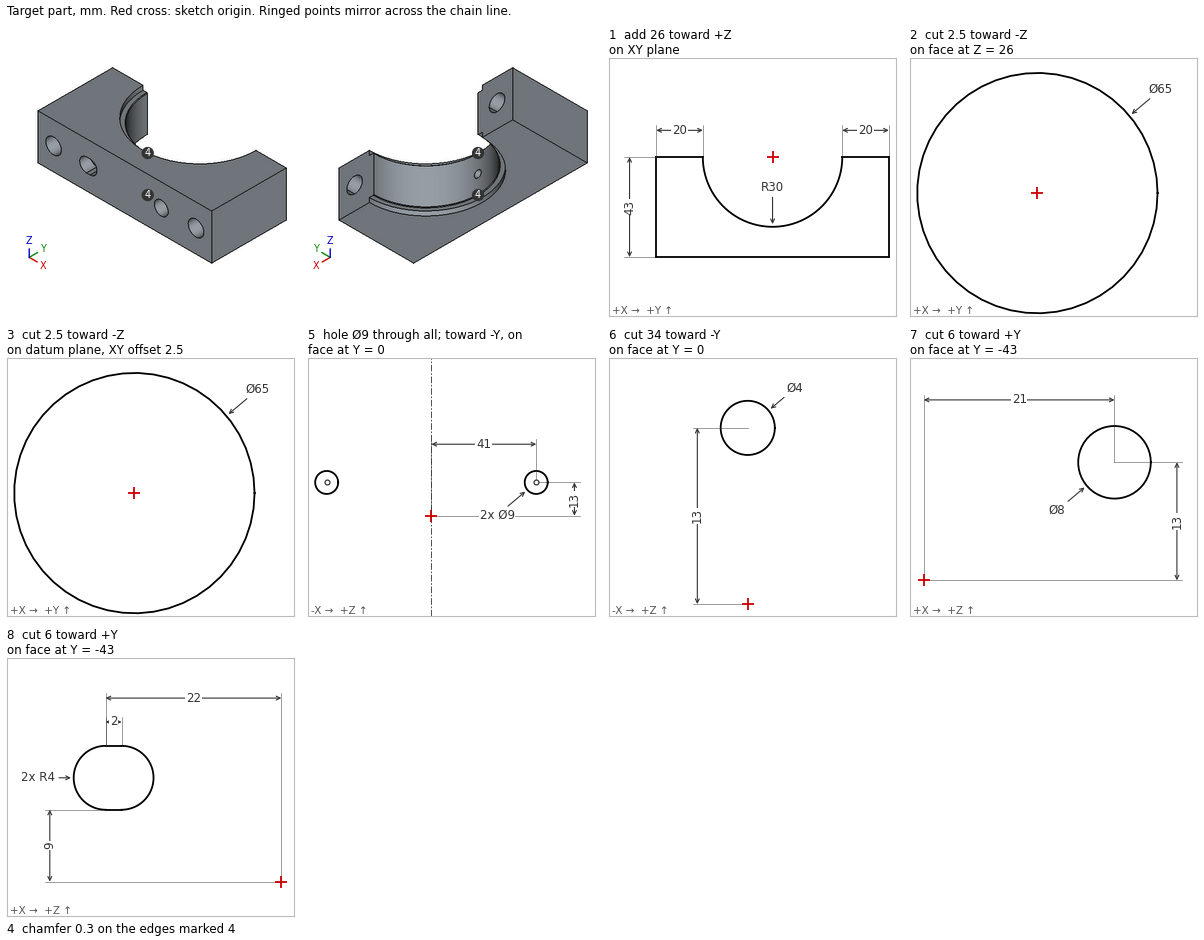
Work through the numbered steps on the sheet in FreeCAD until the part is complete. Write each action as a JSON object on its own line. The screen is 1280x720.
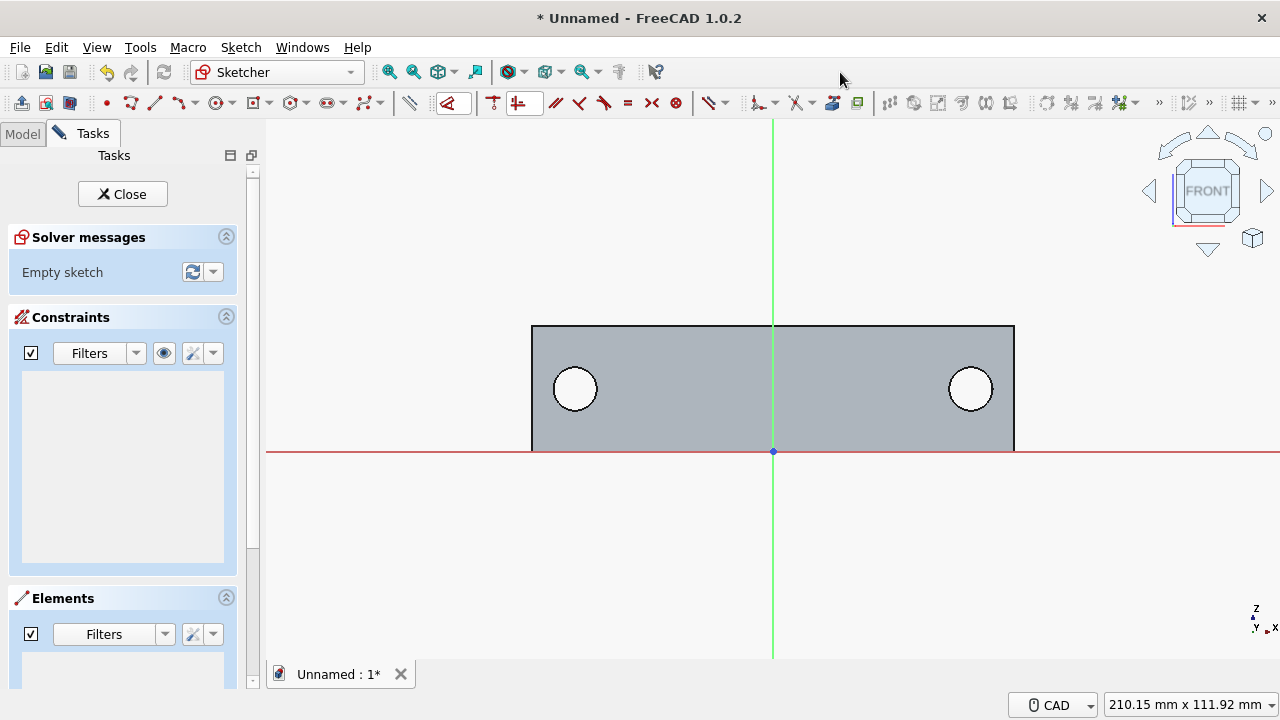
{"action": "scroll", "coordinate": [895, 389], "scroll_direction": "up", "scroll_amount": 11}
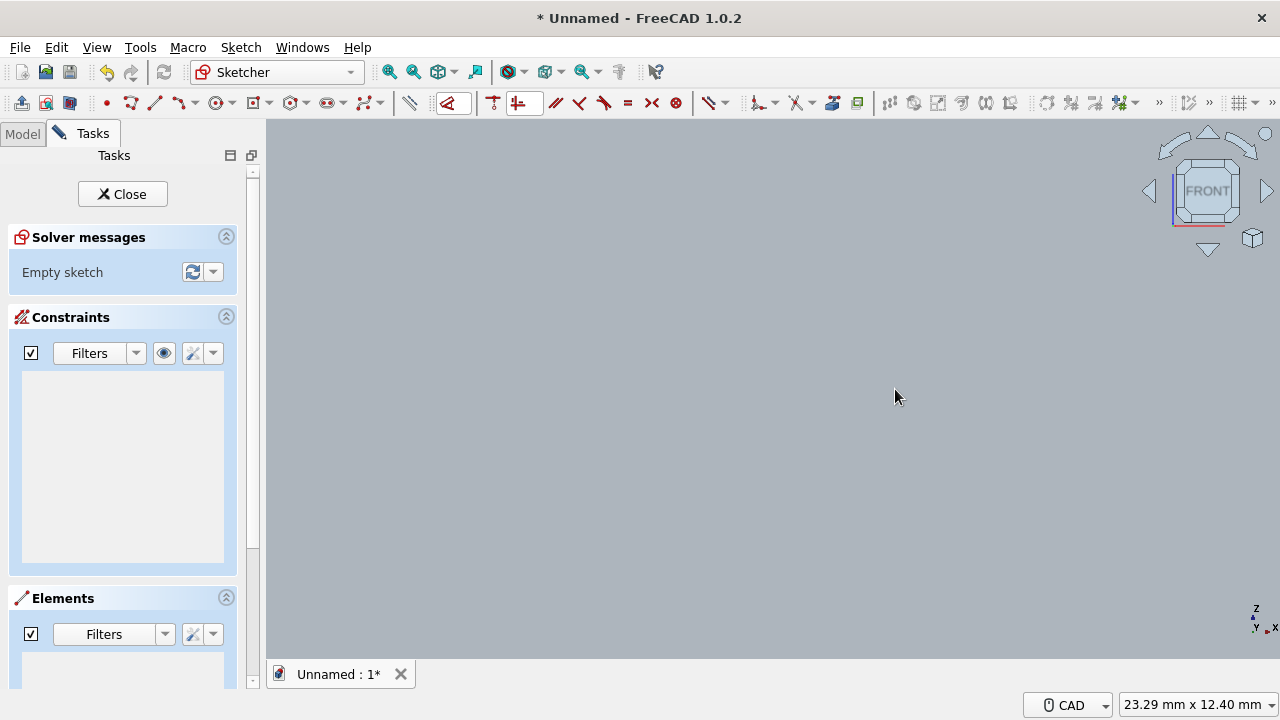
{"action": "left_click", "coordinate": [216, 104]}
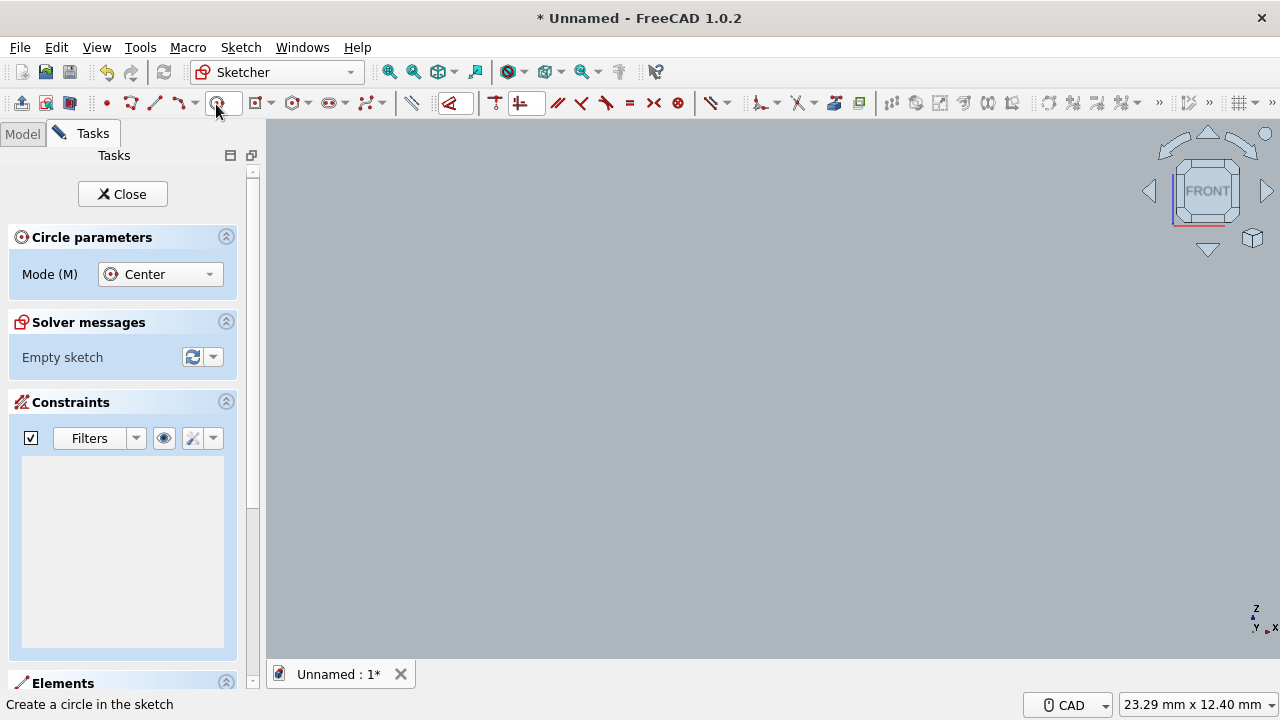
{"action": "left_click", "coordinate": [703, 385]}
{"action": "left_click", "coordinate": [827, 262]}
{"action": "key", "text": "Escape"}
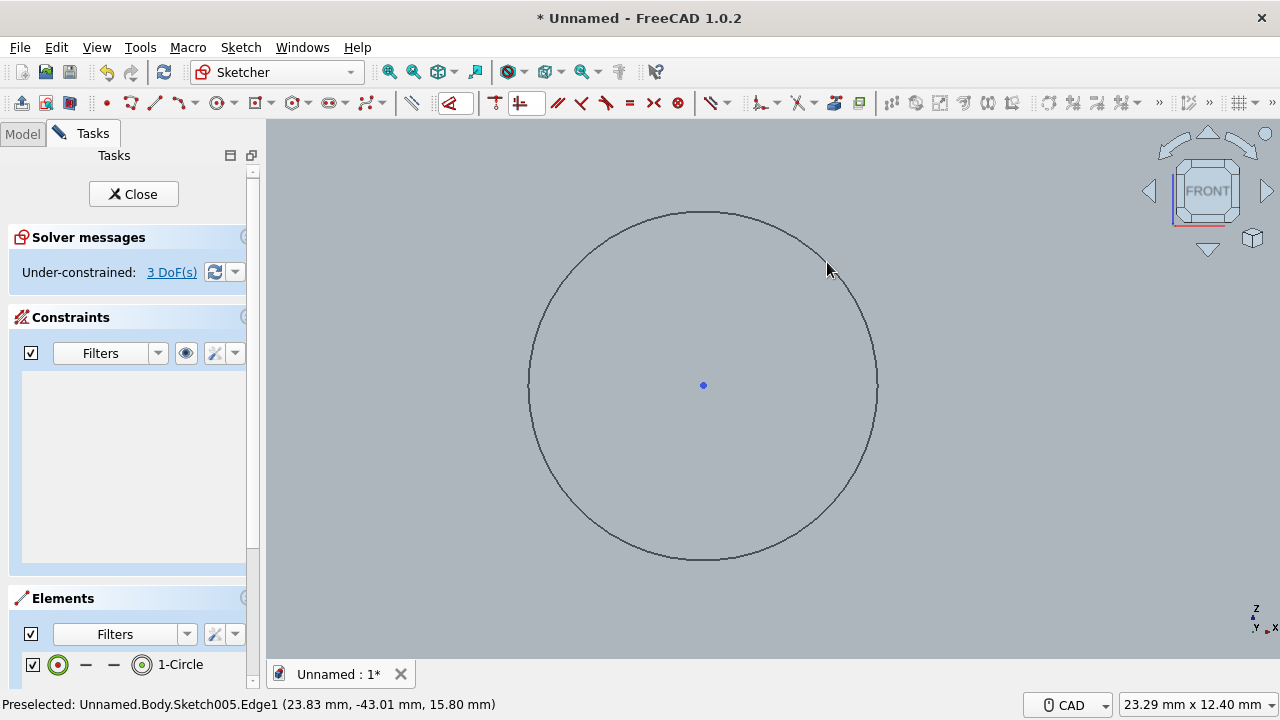
{"action": "left_click", "coordinate": [826, 262]}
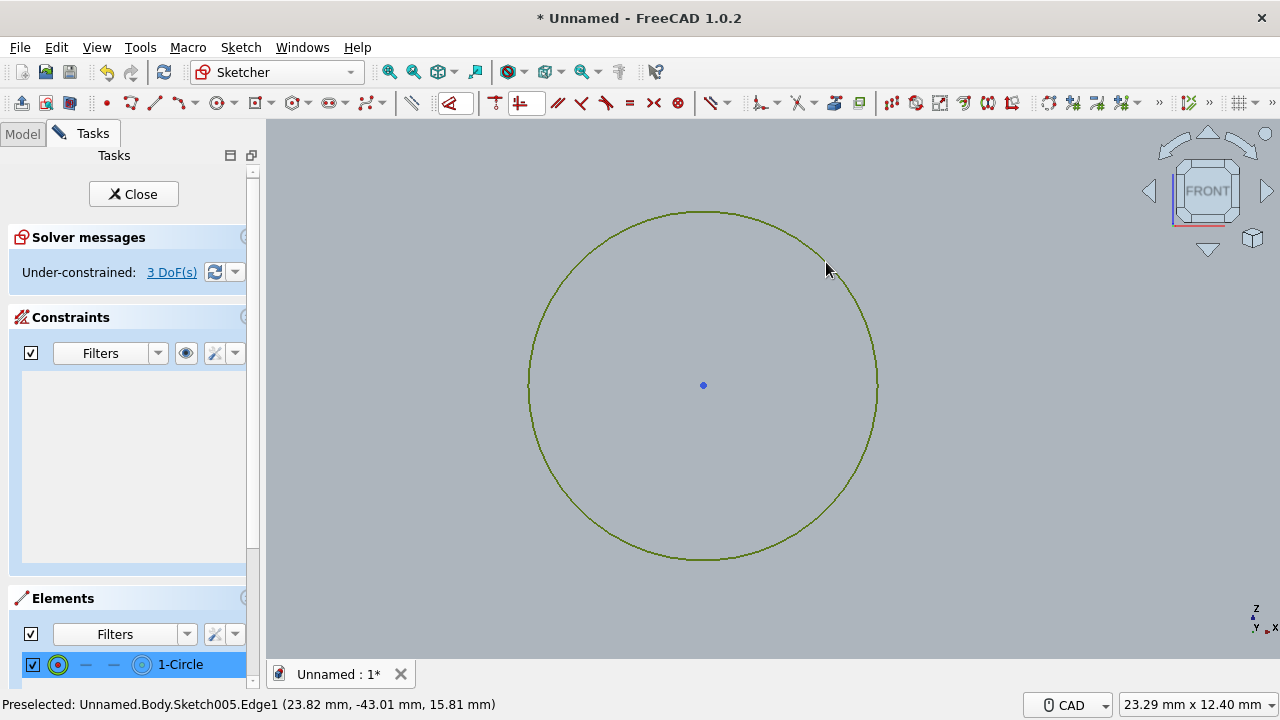
{"action": "key", "text": "k o"}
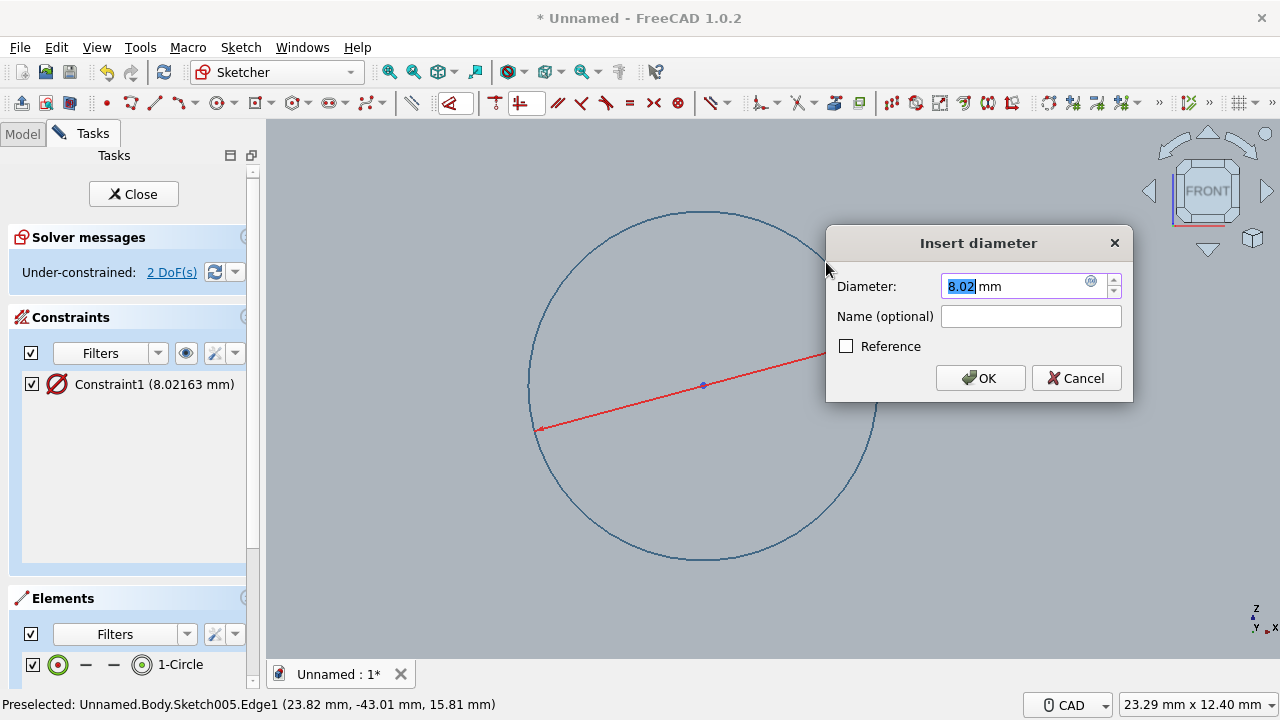
{"action": "type", "text": "8"}
{"action": "key", "text": "Return"}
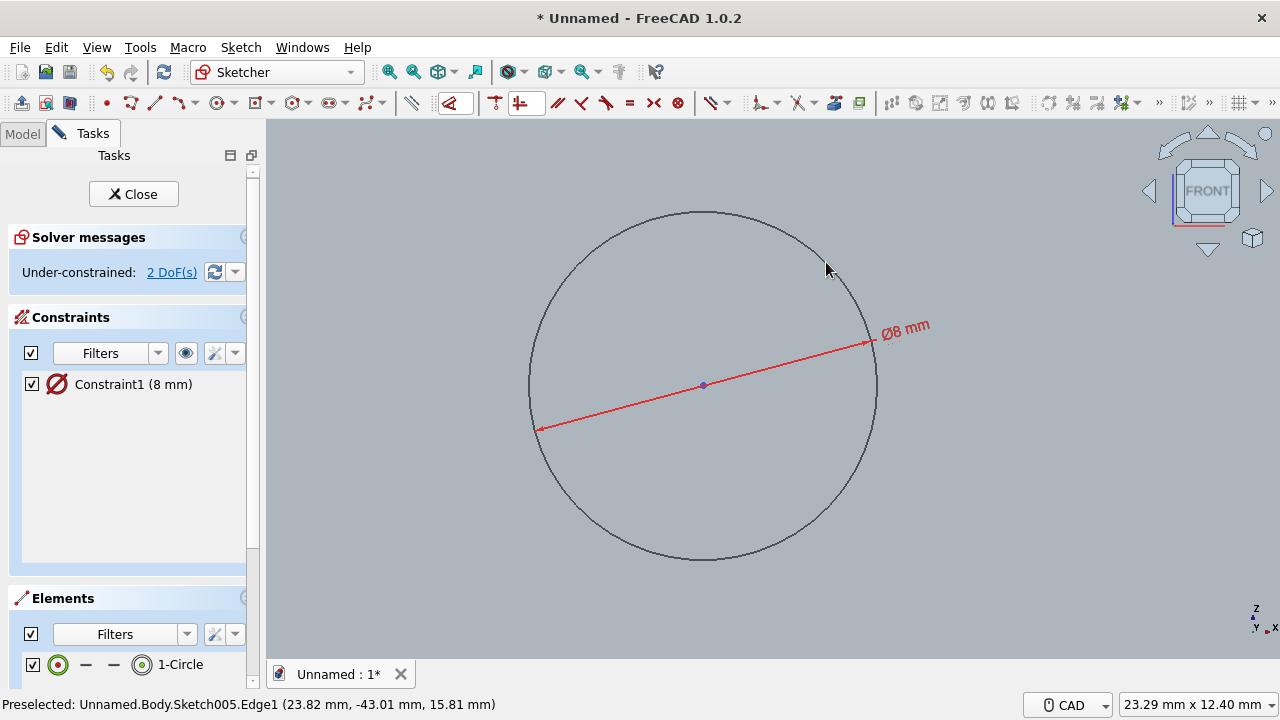
{"action": "left_click", "coordinate": [703, 386]}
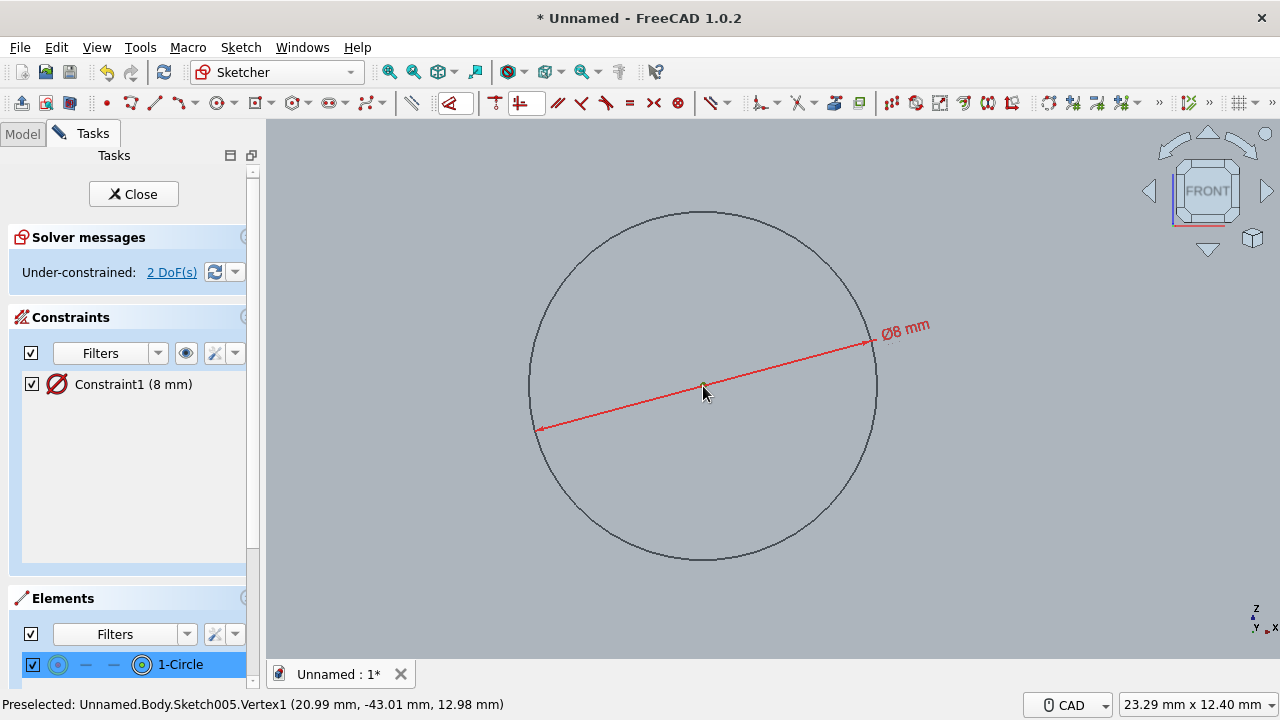
{"action": "left_click", "coordinate": [468, 104]}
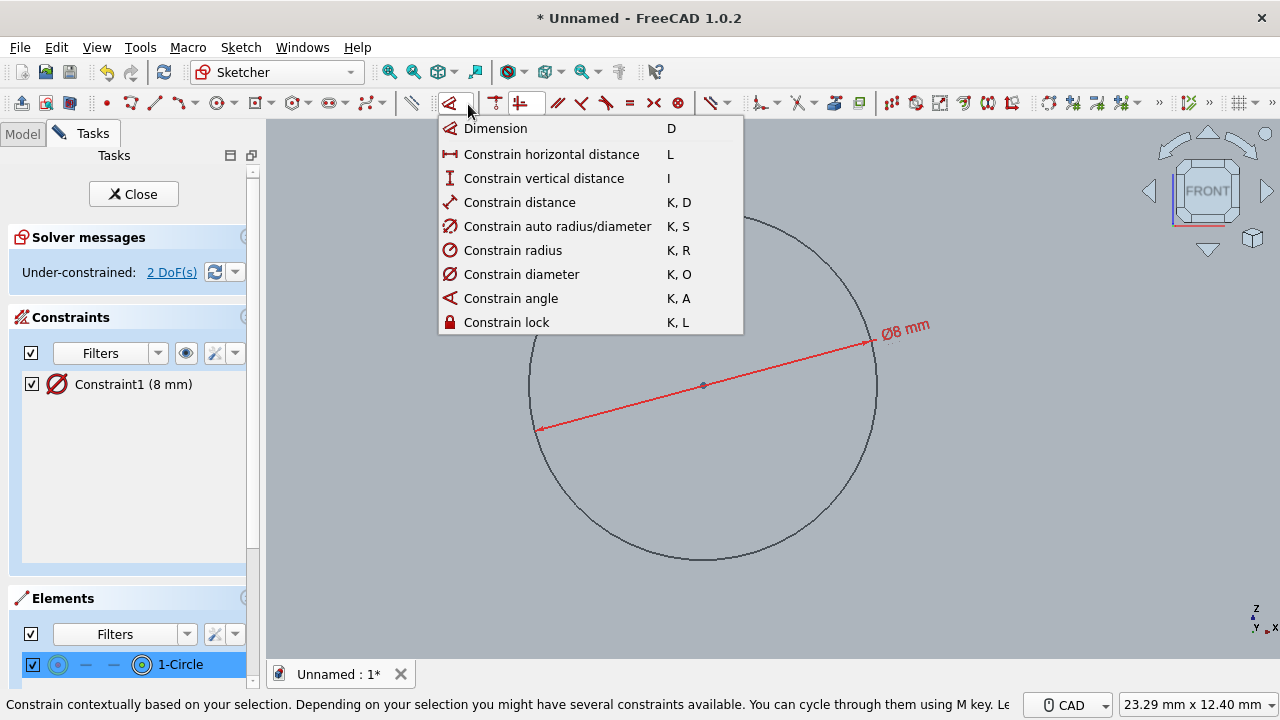
{"action": "left_click", "coordinate": [591, 154]}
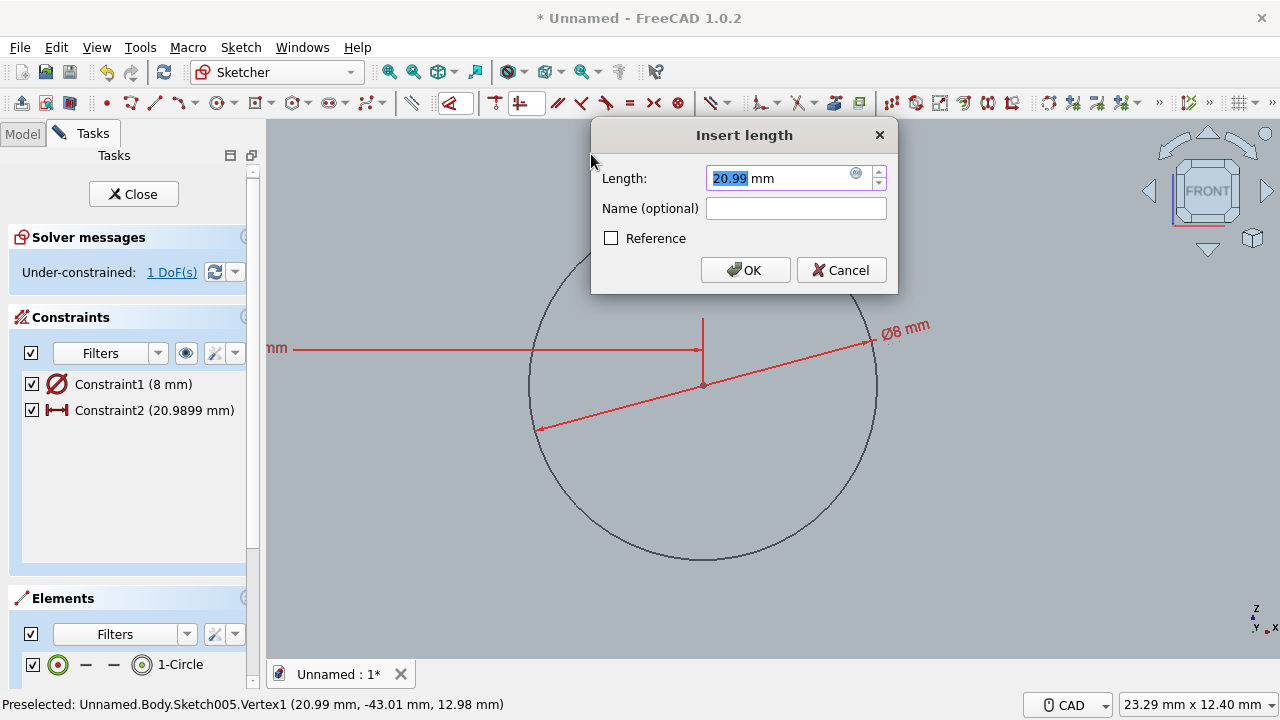
{"action": "type", "text": "21"}
{"action": "key", "text": "Return"}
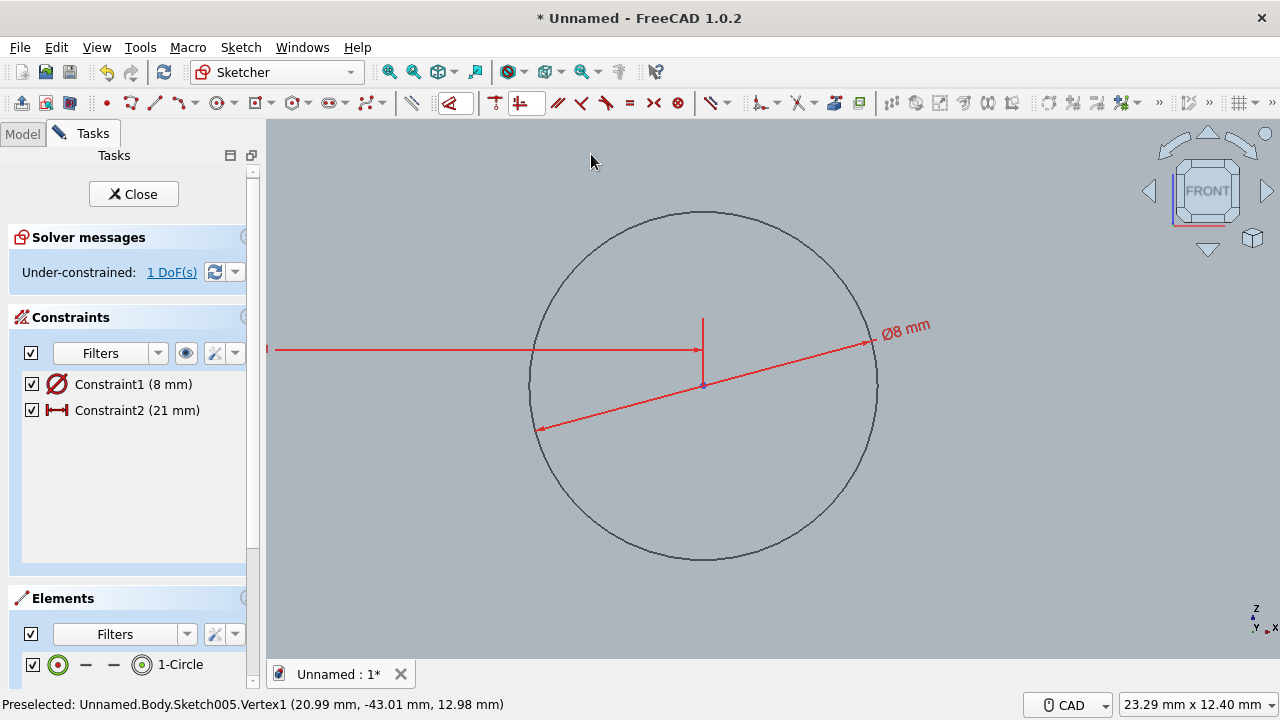
{"action": "left_click", "coordinate": [703, 386]}